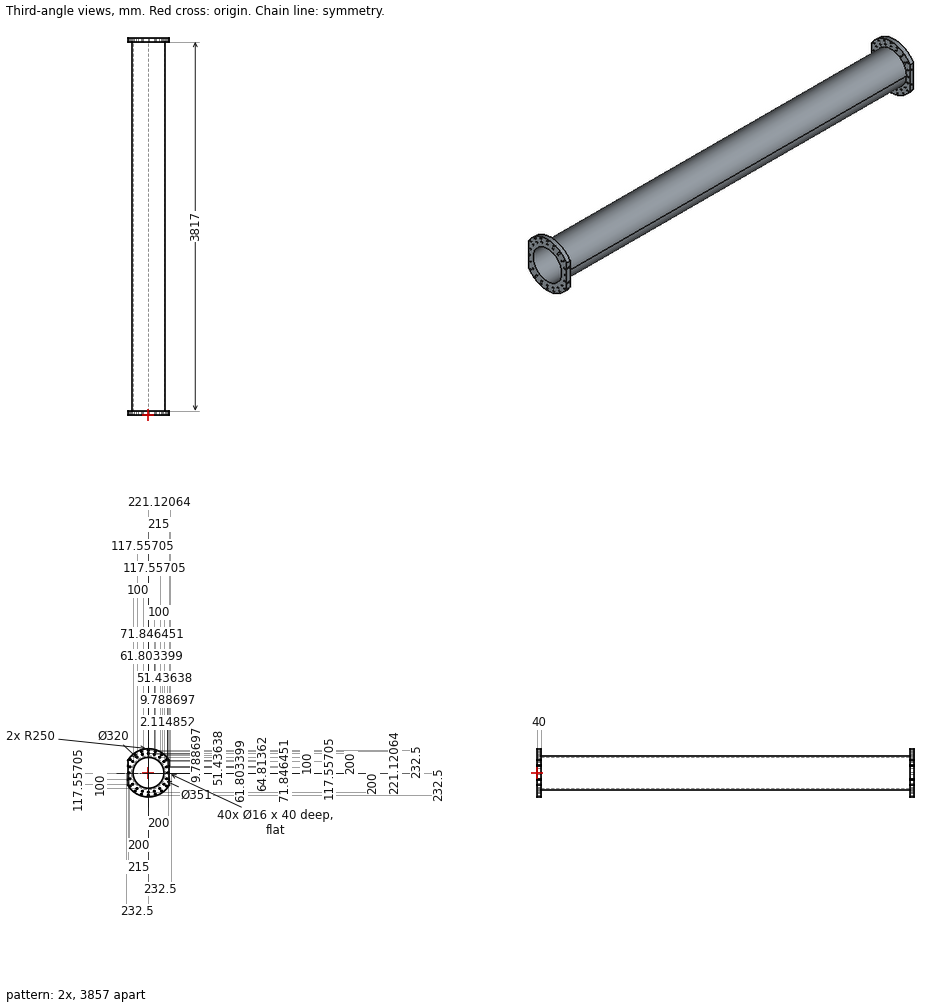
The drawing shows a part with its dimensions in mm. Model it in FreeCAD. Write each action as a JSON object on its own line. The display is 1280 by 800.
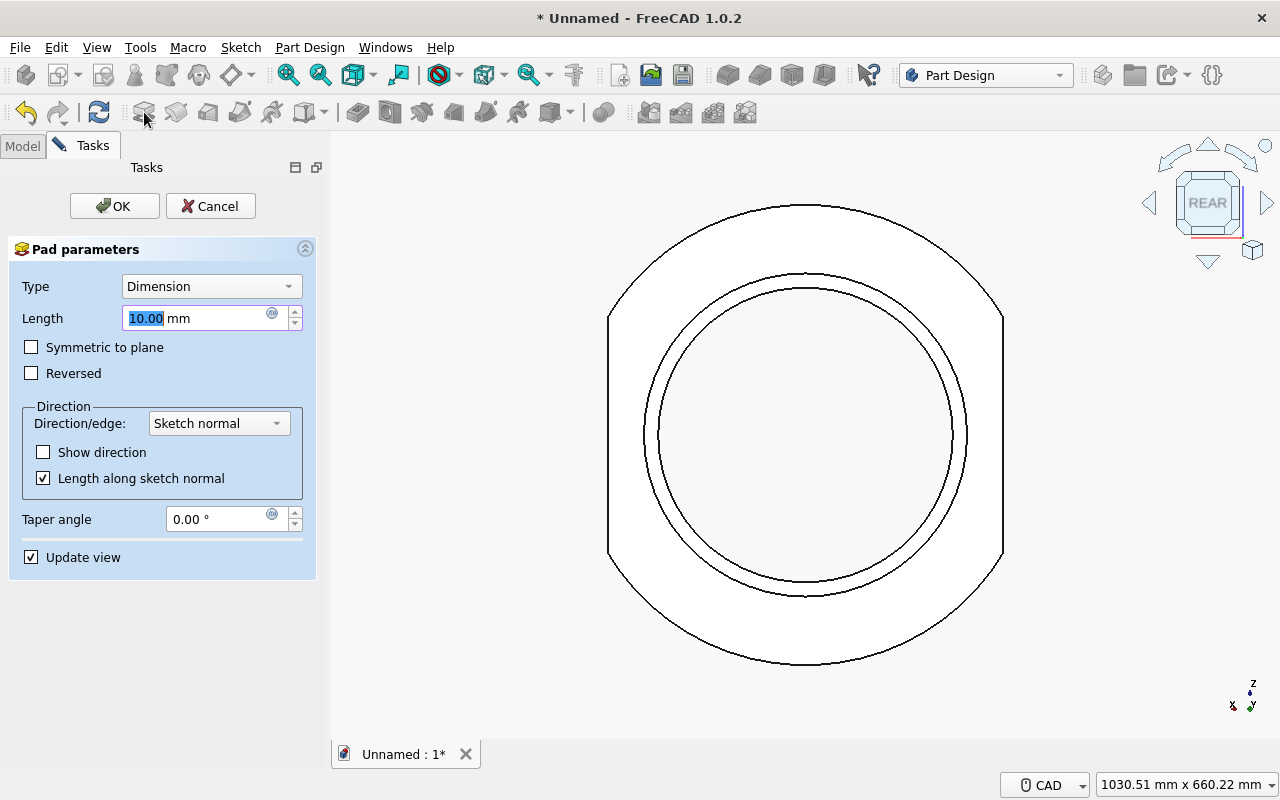
{"action": "type", "text": "3817"}
{"action": "key", "text": "Tab"}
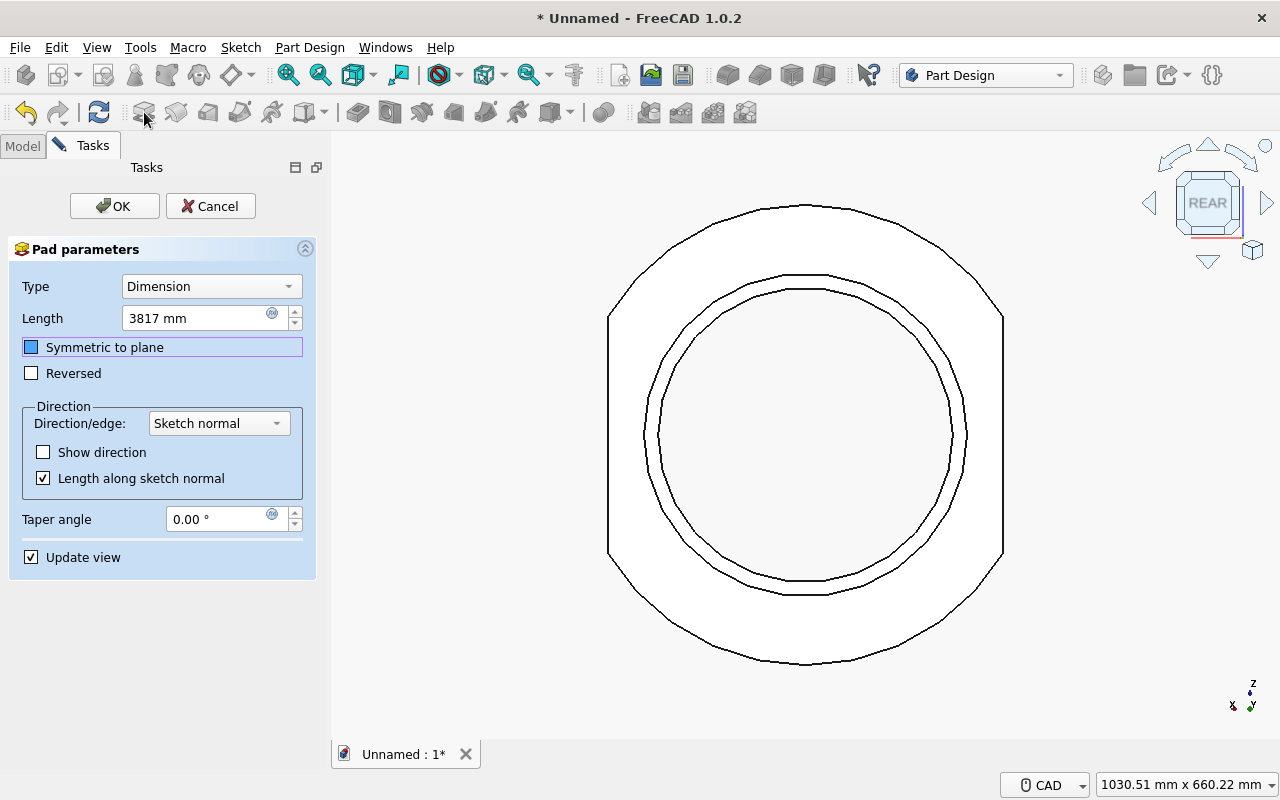
{"action": "left_click", "coordinate": [115, 206]}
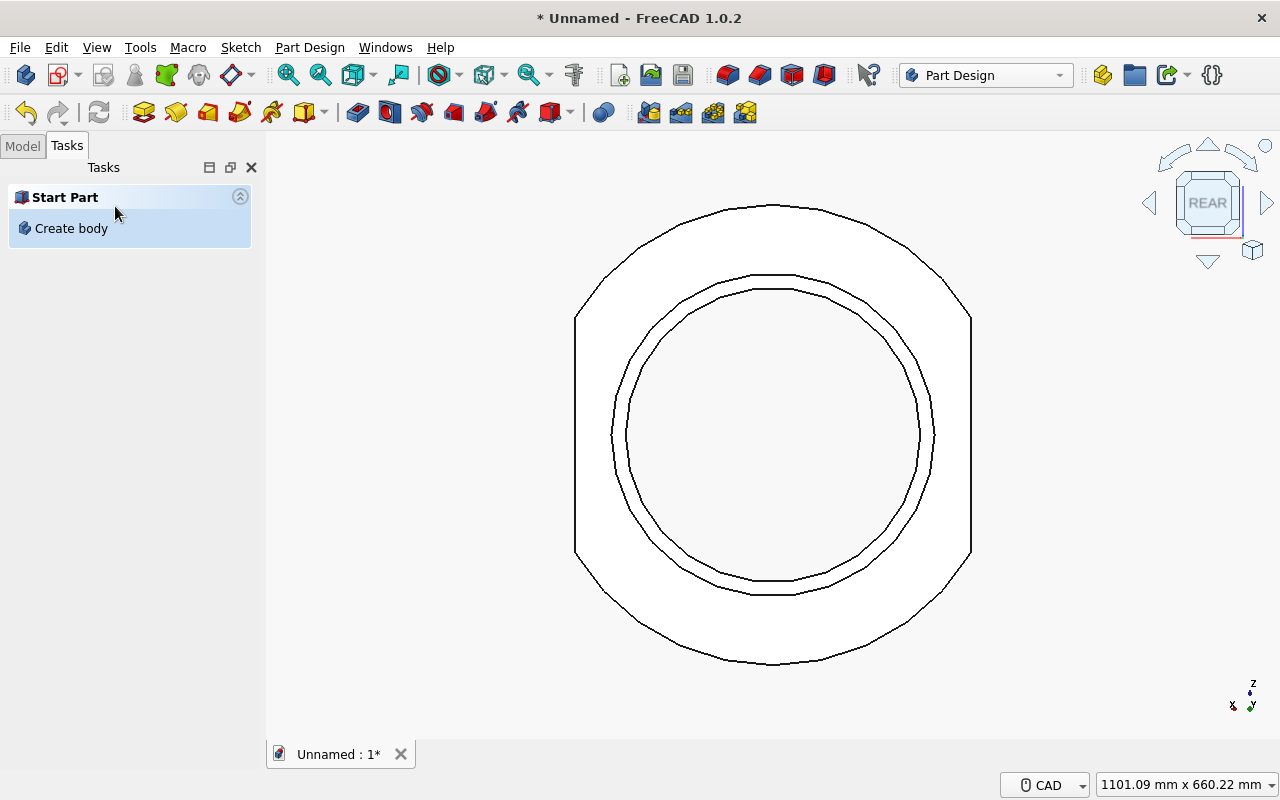
{"action": "left_click", "coordinate": [773, 237]}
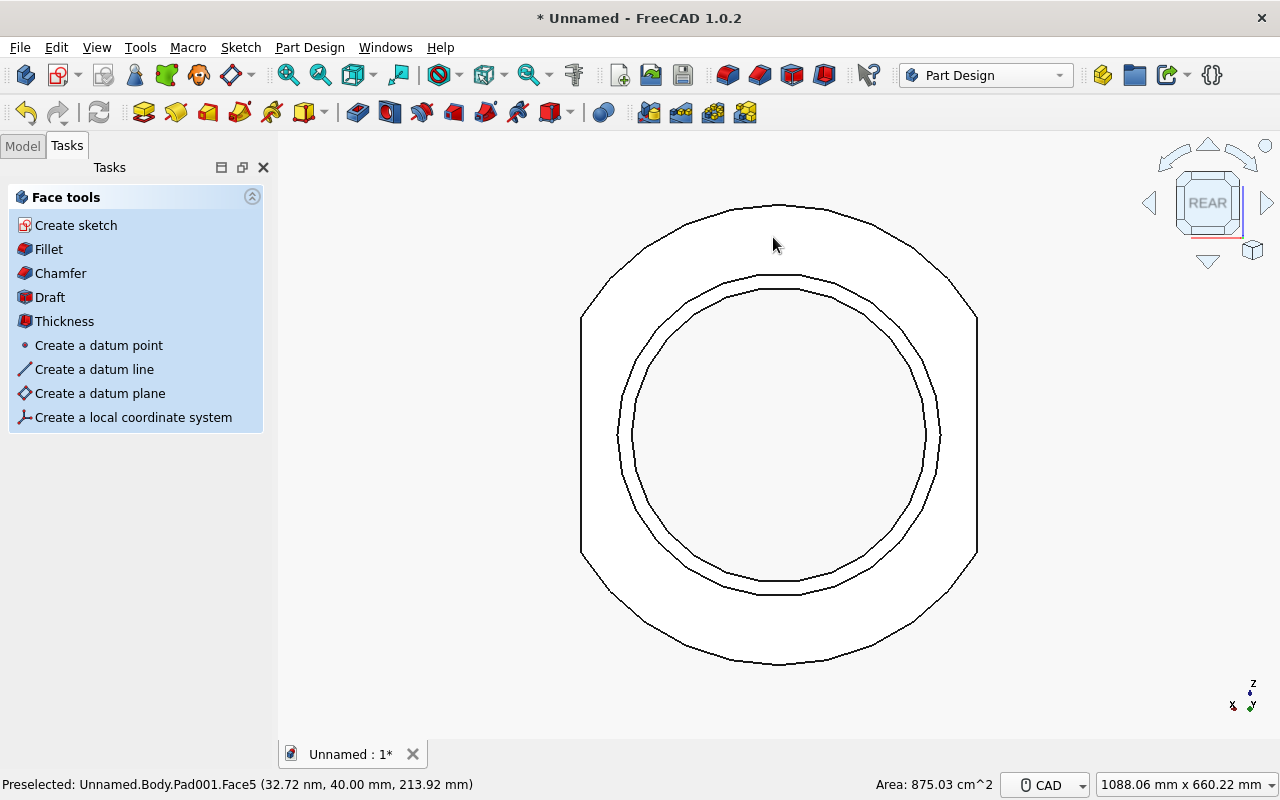
{"action": "left_click", "coordinate": [58, 76]}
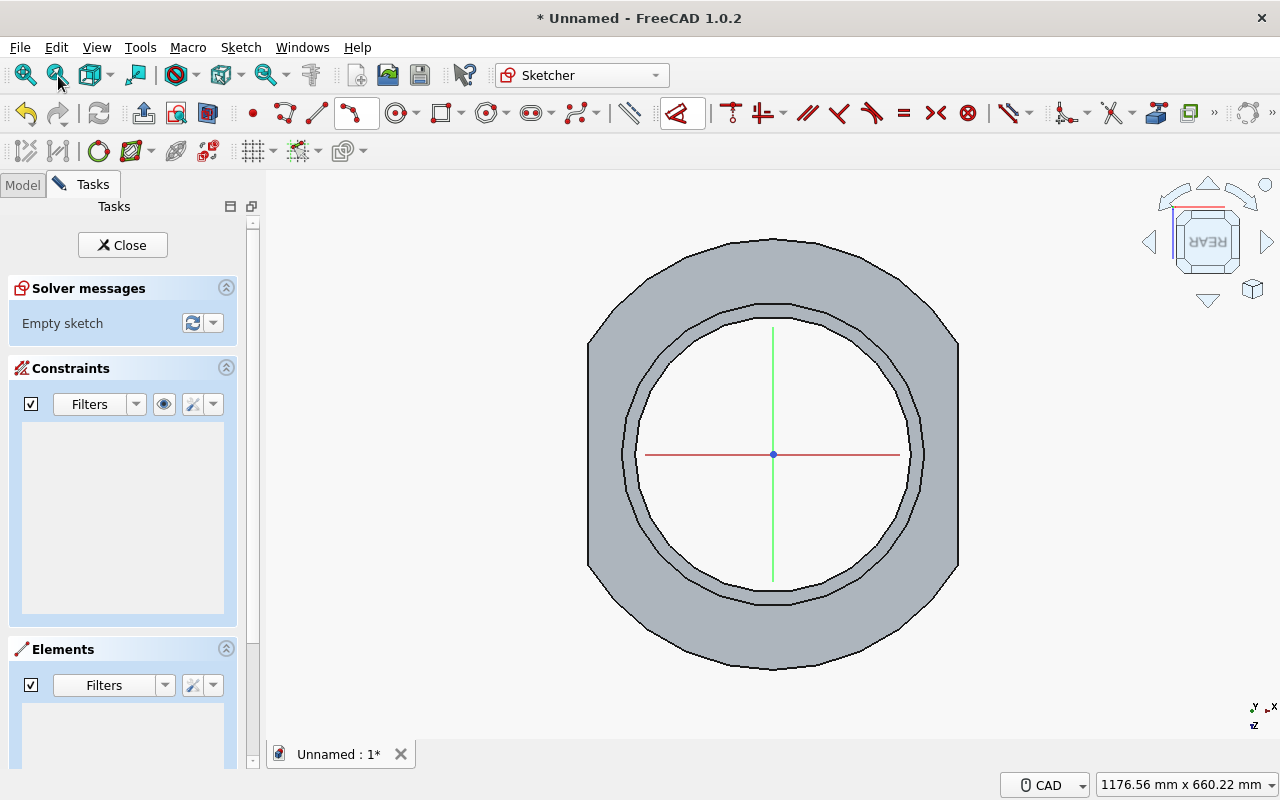
{"action": "left_click", "coordinate": [396, 114]}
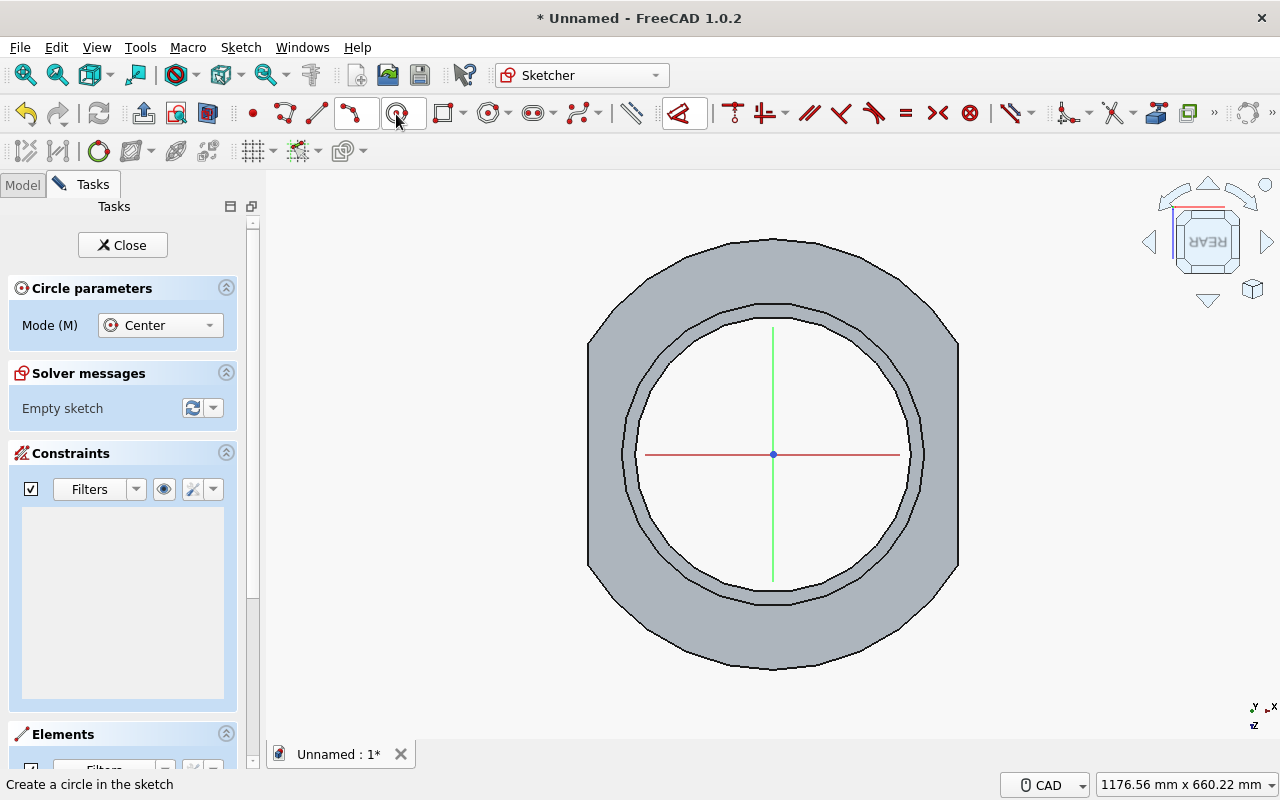
{"action": "scroll", "coordinate": [945, 454], "scroll_direction": "up", "scroll_amount": 6}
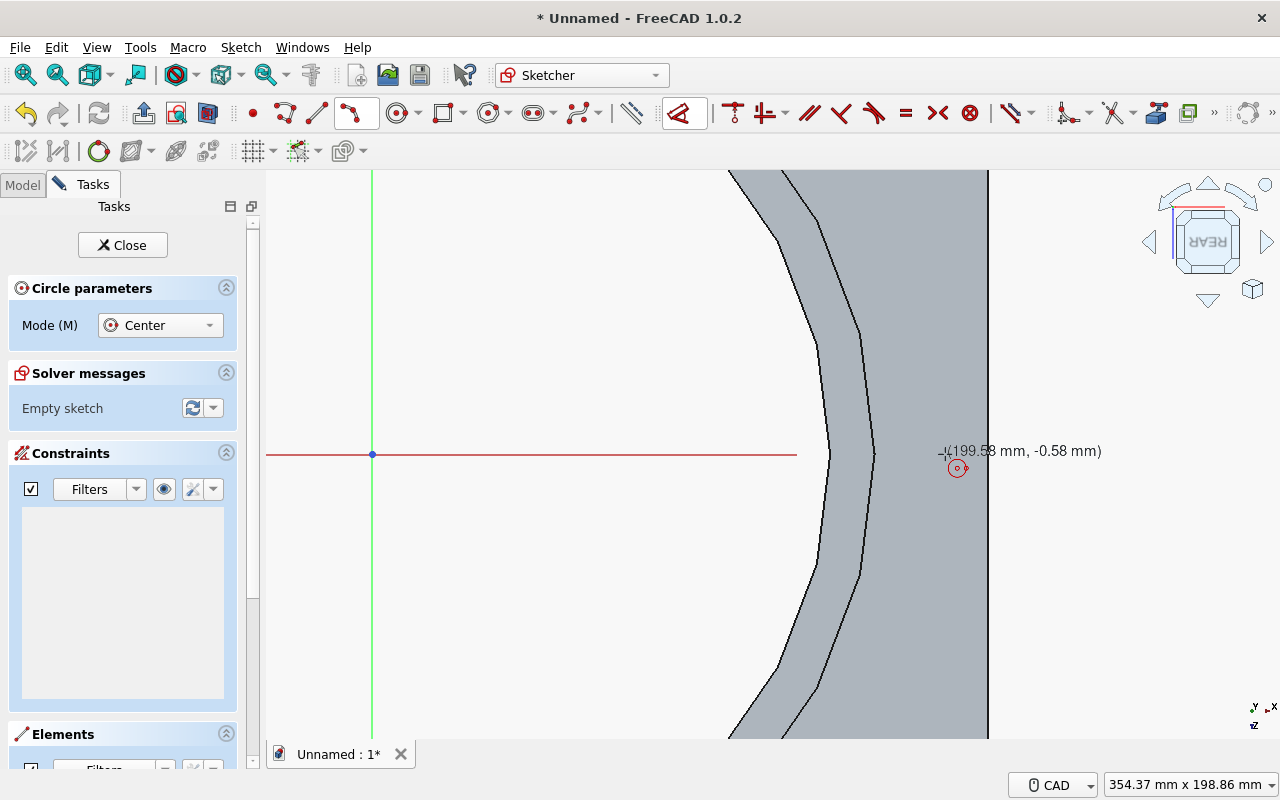
{"action": "left_click", "coordinate": [945, 454]}
{"action": "mouse_move", "coordinate": [961, 438]}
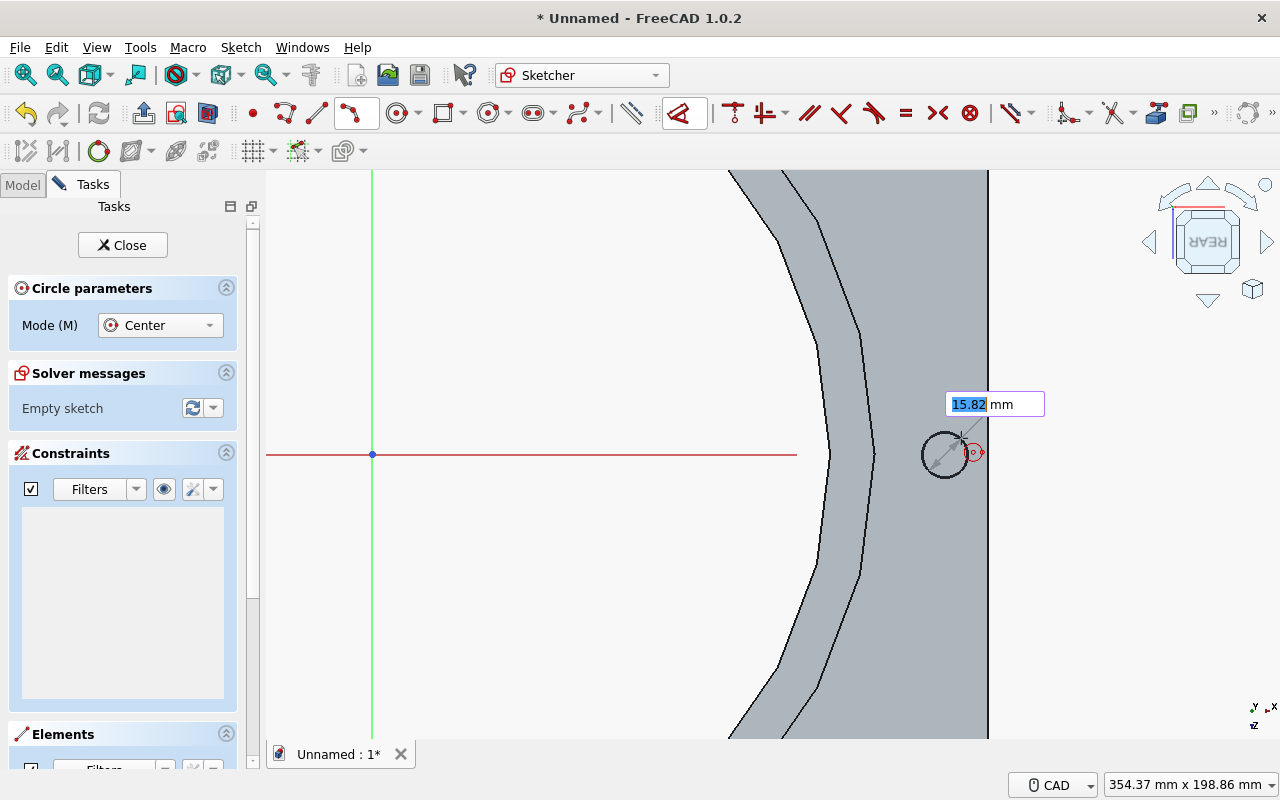
{"action": "type", "text": "16"}
{"action": "key", "text": "Return"}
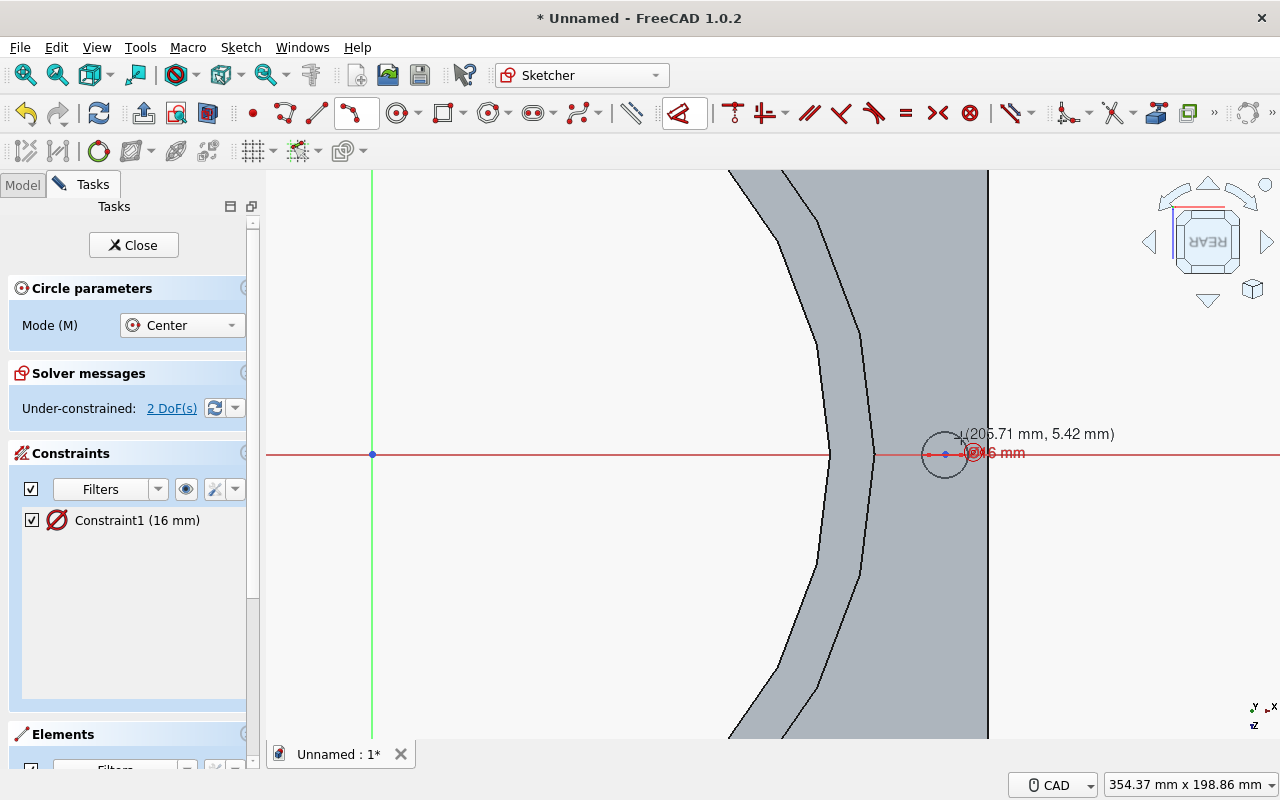
{"action": "left_click", "coordinate": [917, 631]}
{"action": "mouse_move", "coordinate": [933, 615]}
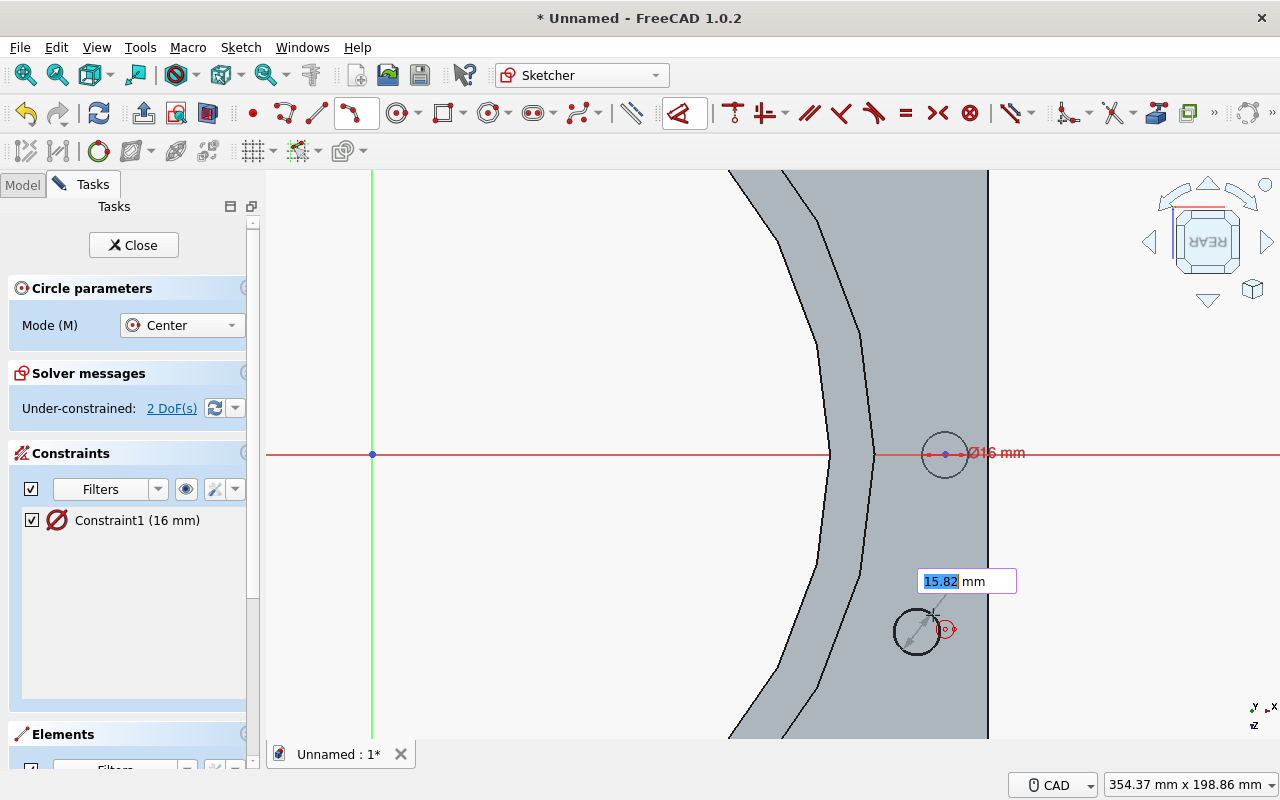
{"action": "type", "text": "16"}
{"action": "key", "text": "Return"}